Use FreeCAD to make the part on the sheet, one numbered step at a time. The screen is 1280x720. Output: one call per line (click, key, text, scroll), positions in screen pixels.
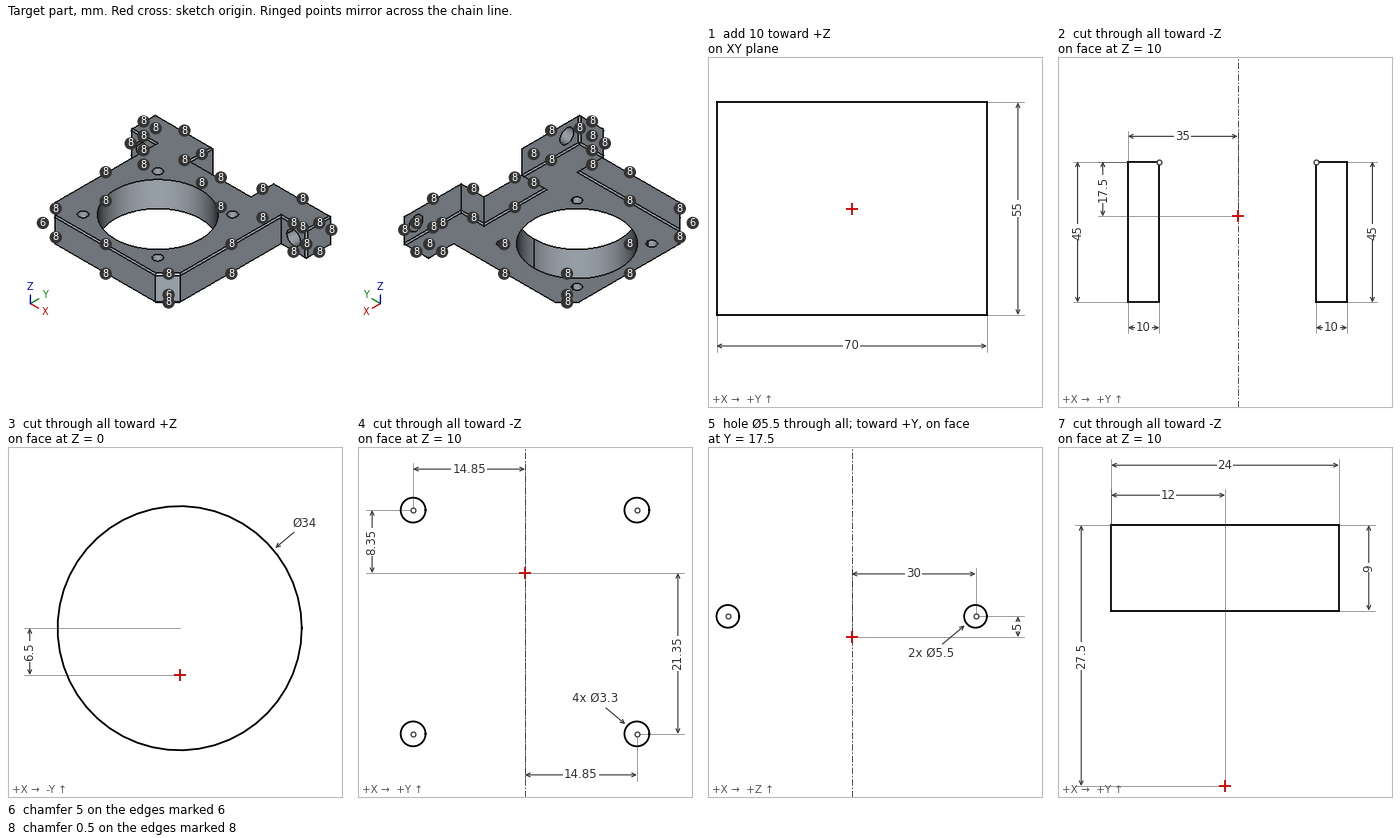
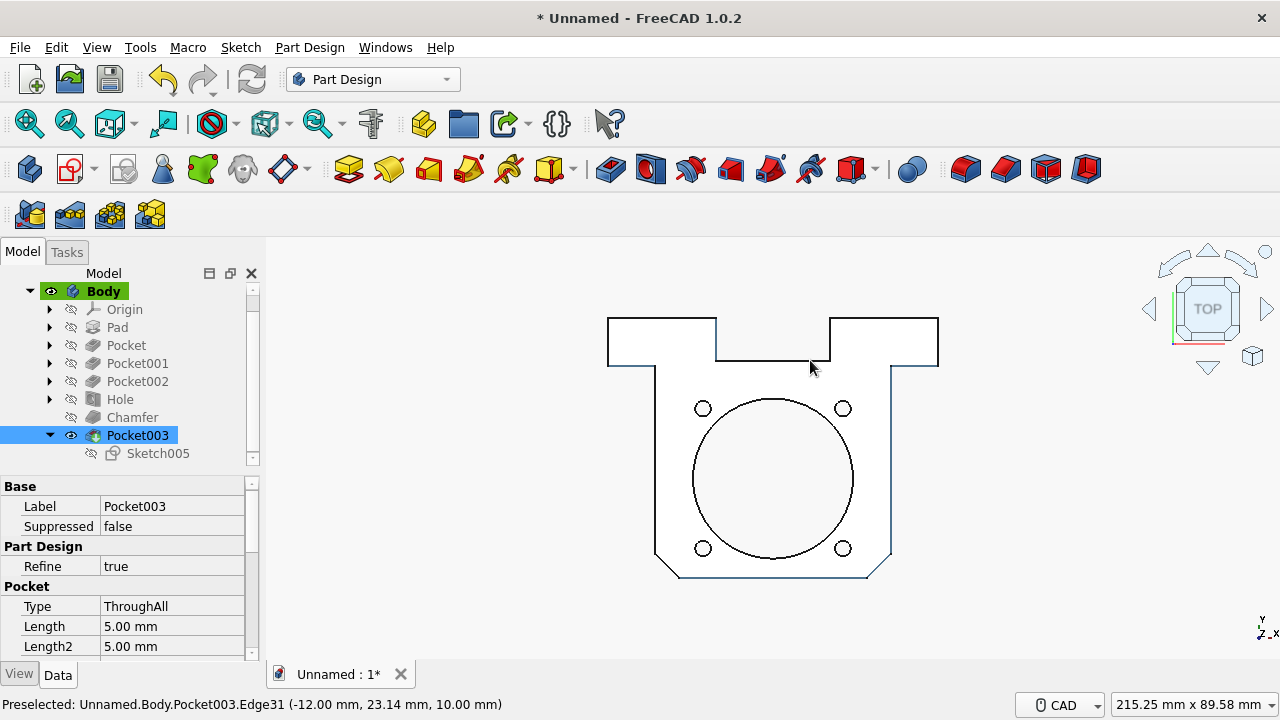
click(773, 360, ctrl)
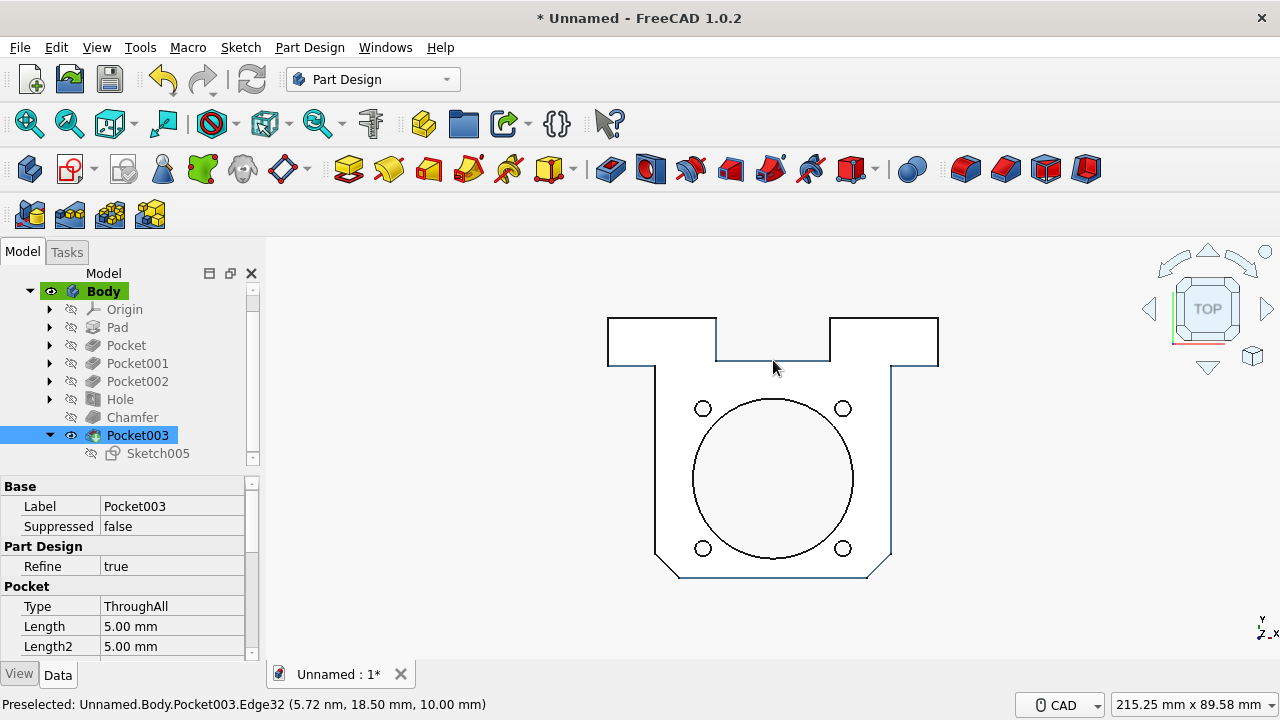
click(830, 339, ctrl)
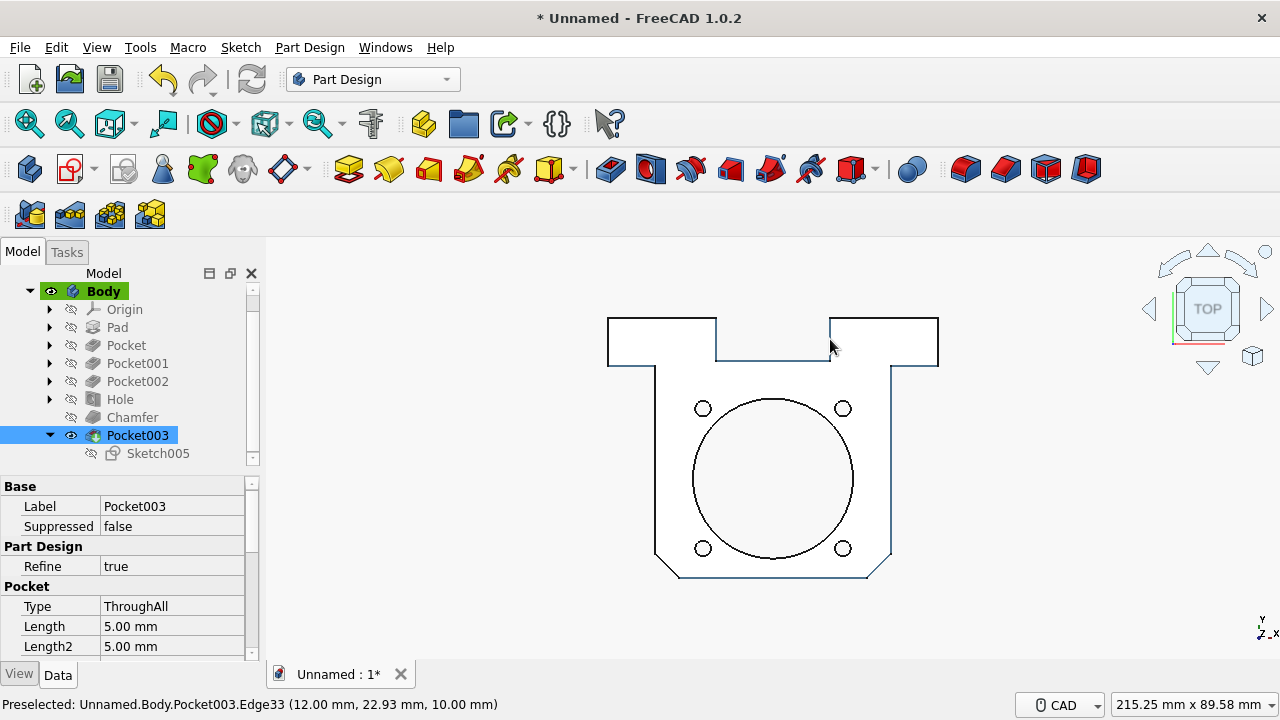
click(884, 317, ctrl)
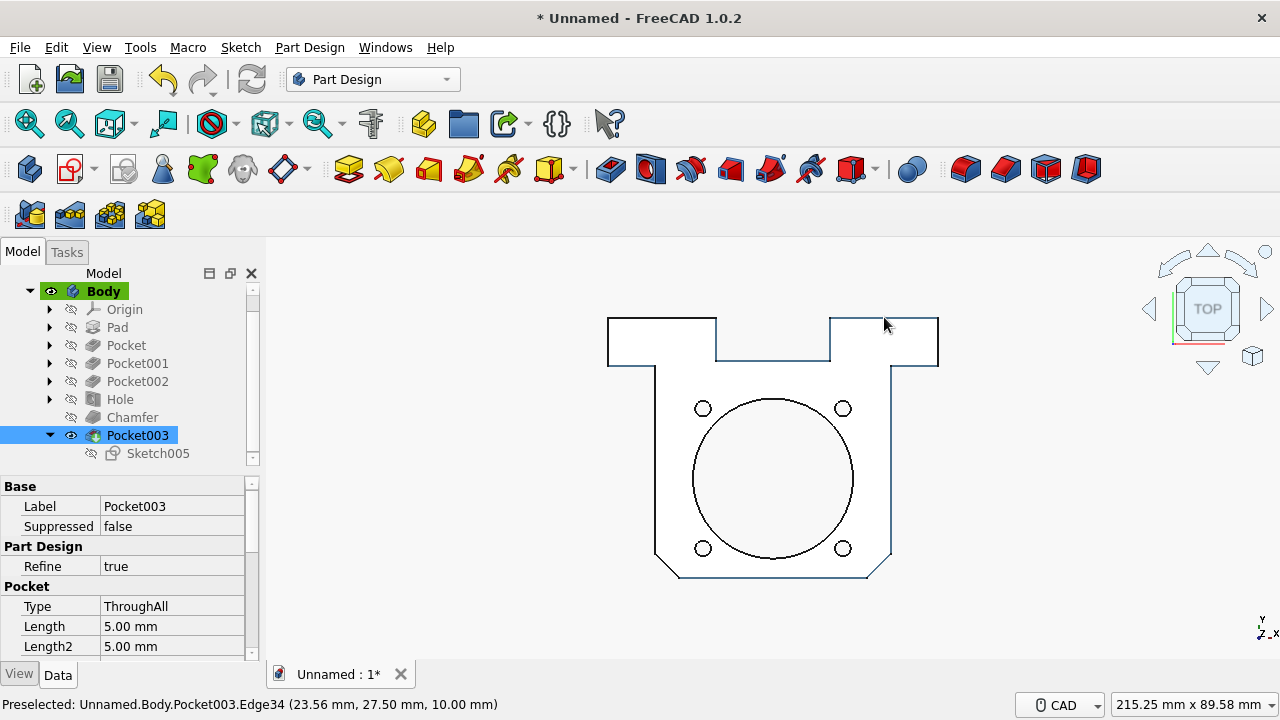
click(655, 459, ctrl)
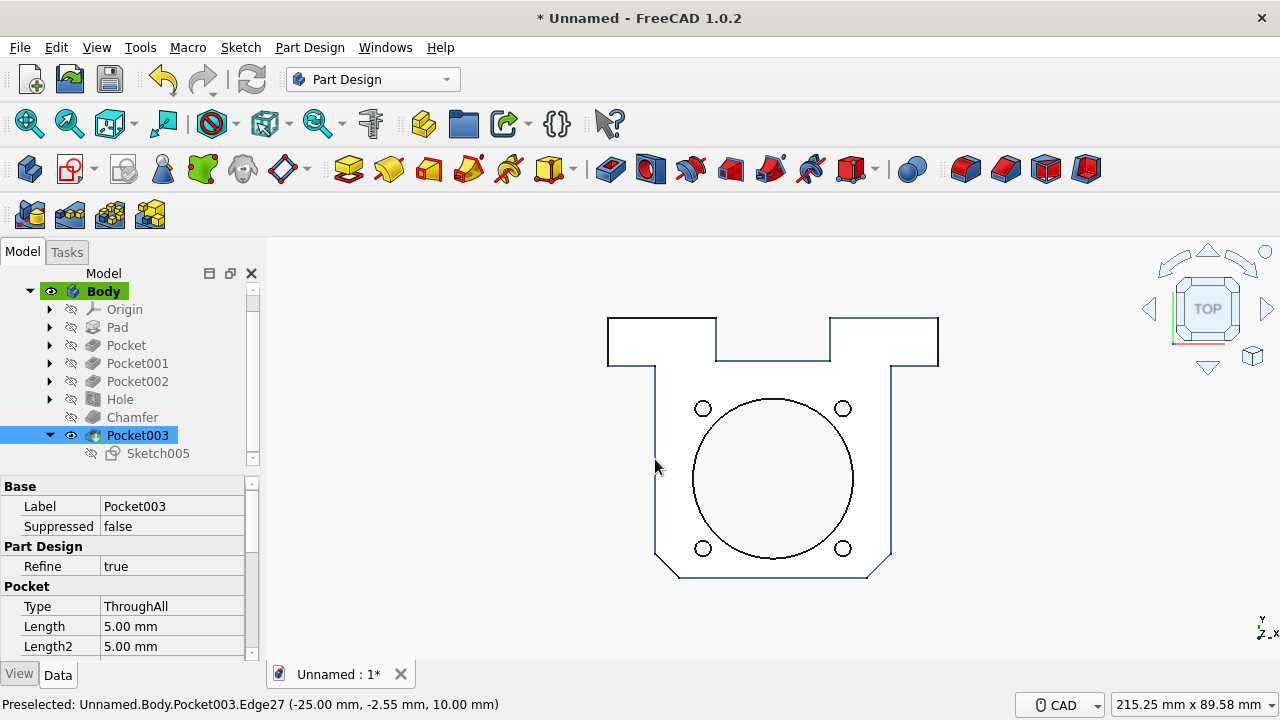
click(667, 565, ctrl)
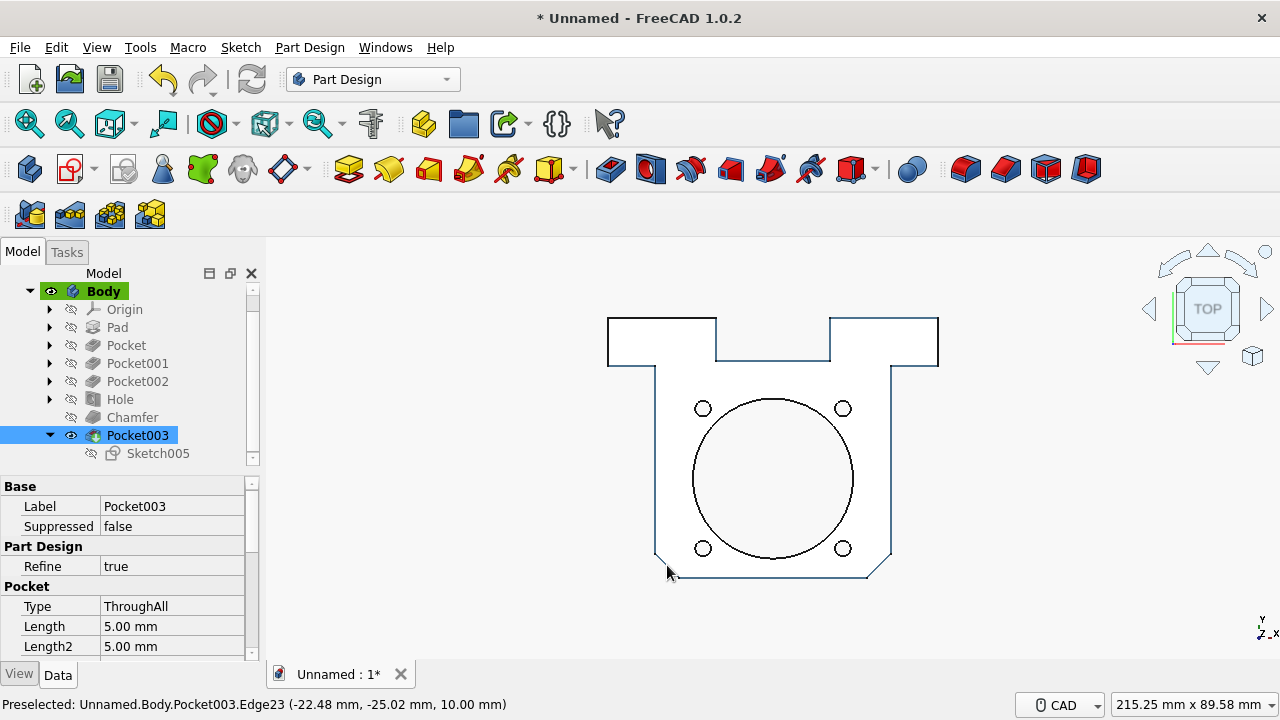
click(662, 317, ctrl)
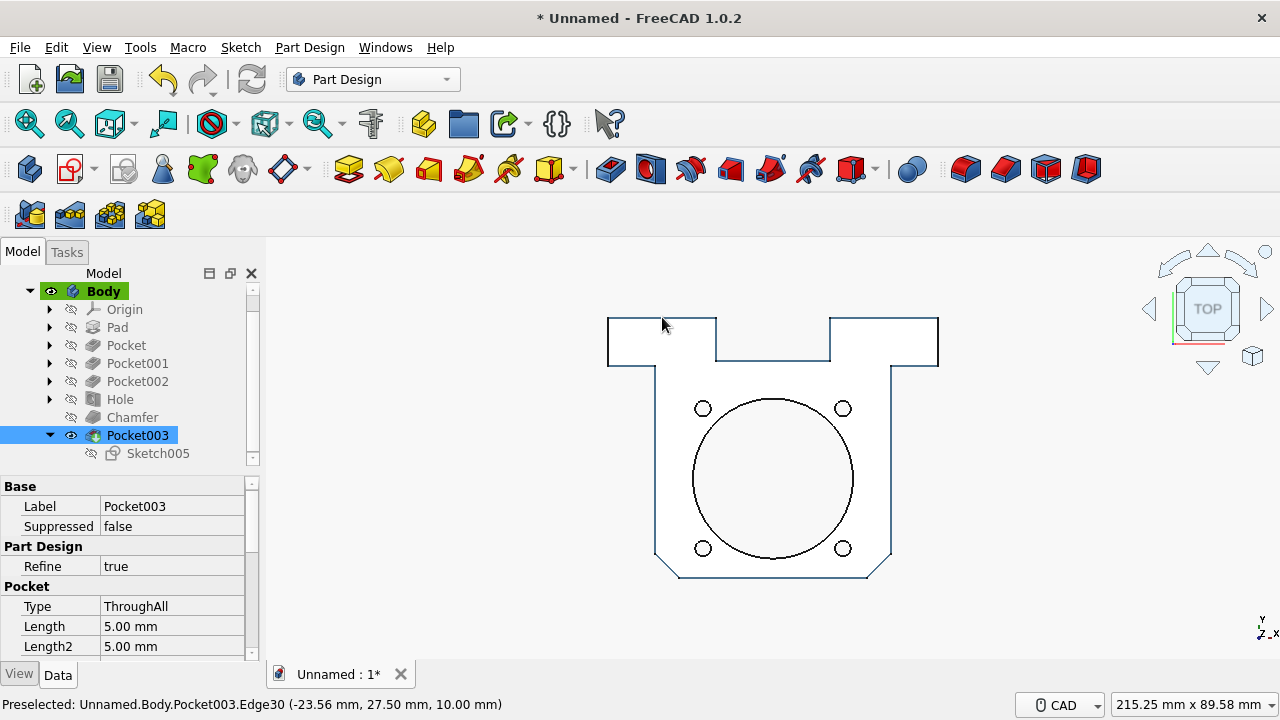
key(0)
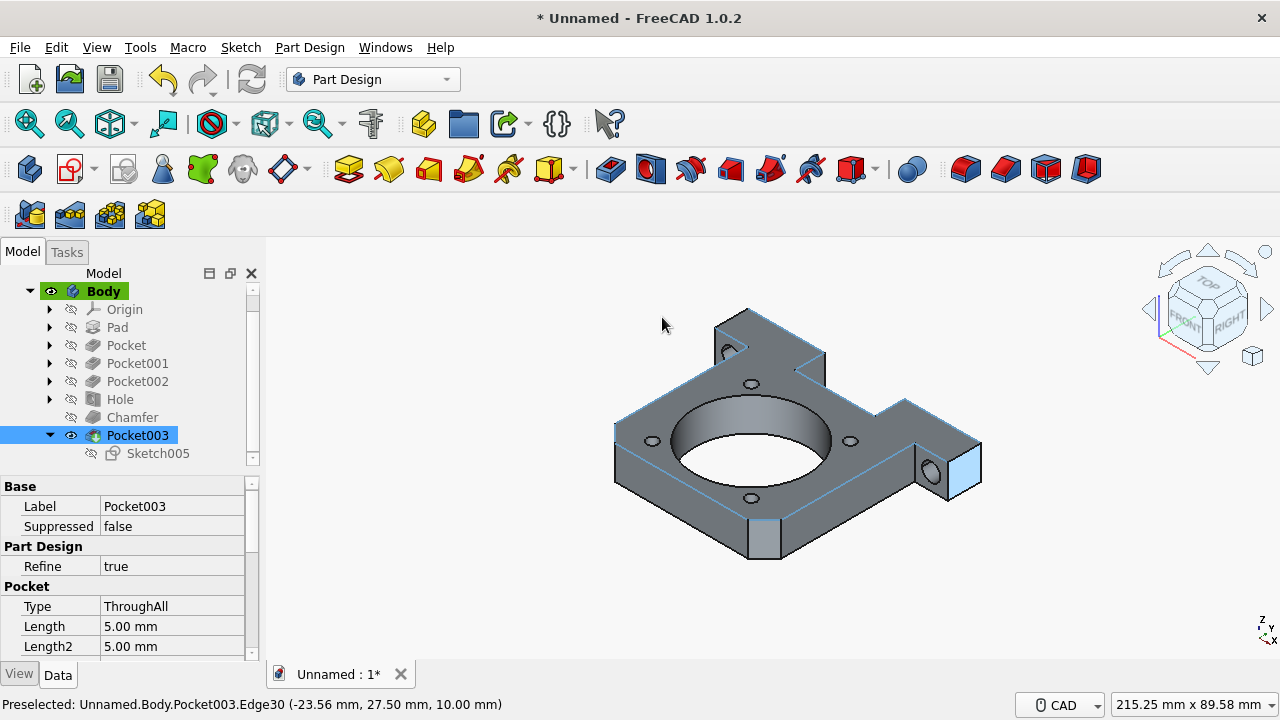
key(1)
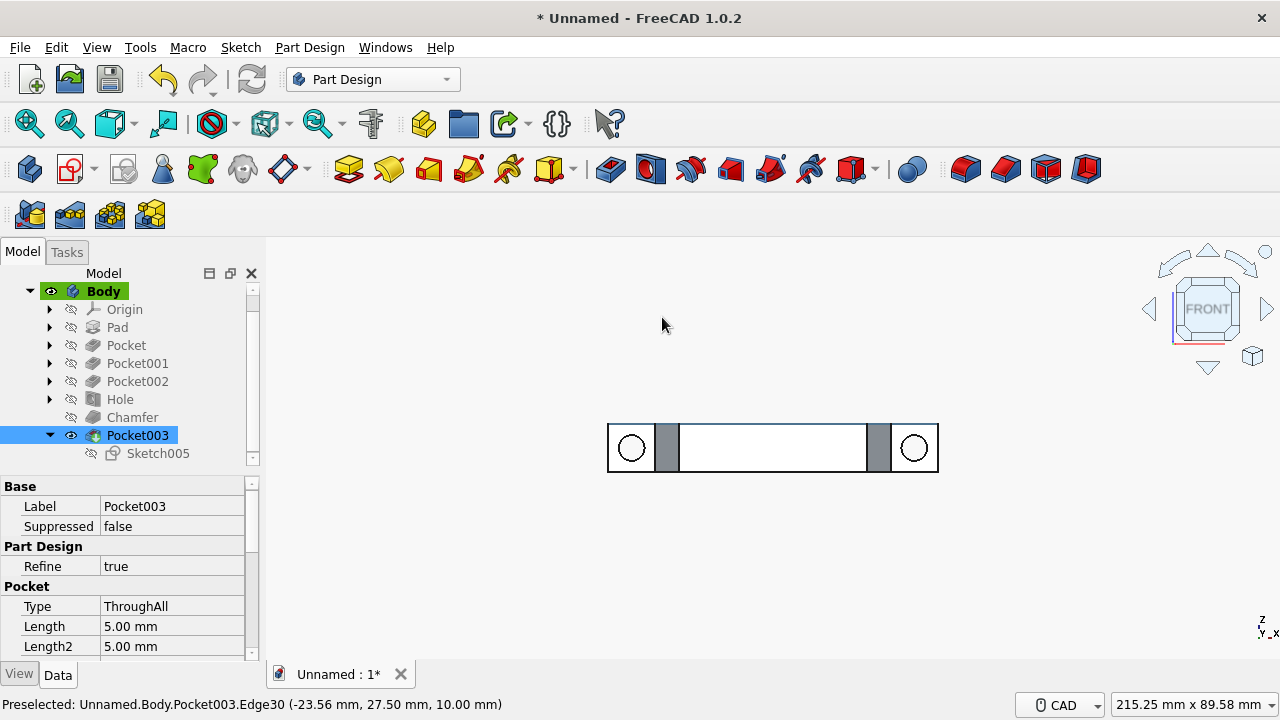
key(v)
key(f)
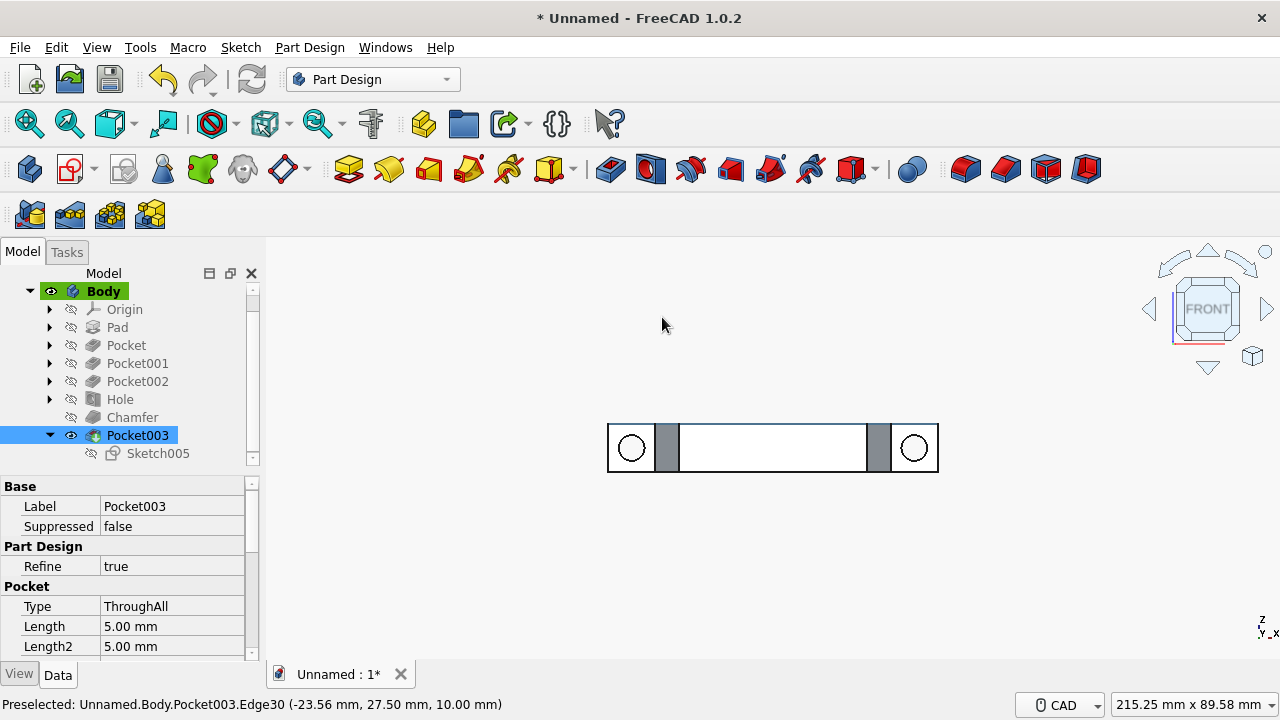
click(632, 471, ctrl)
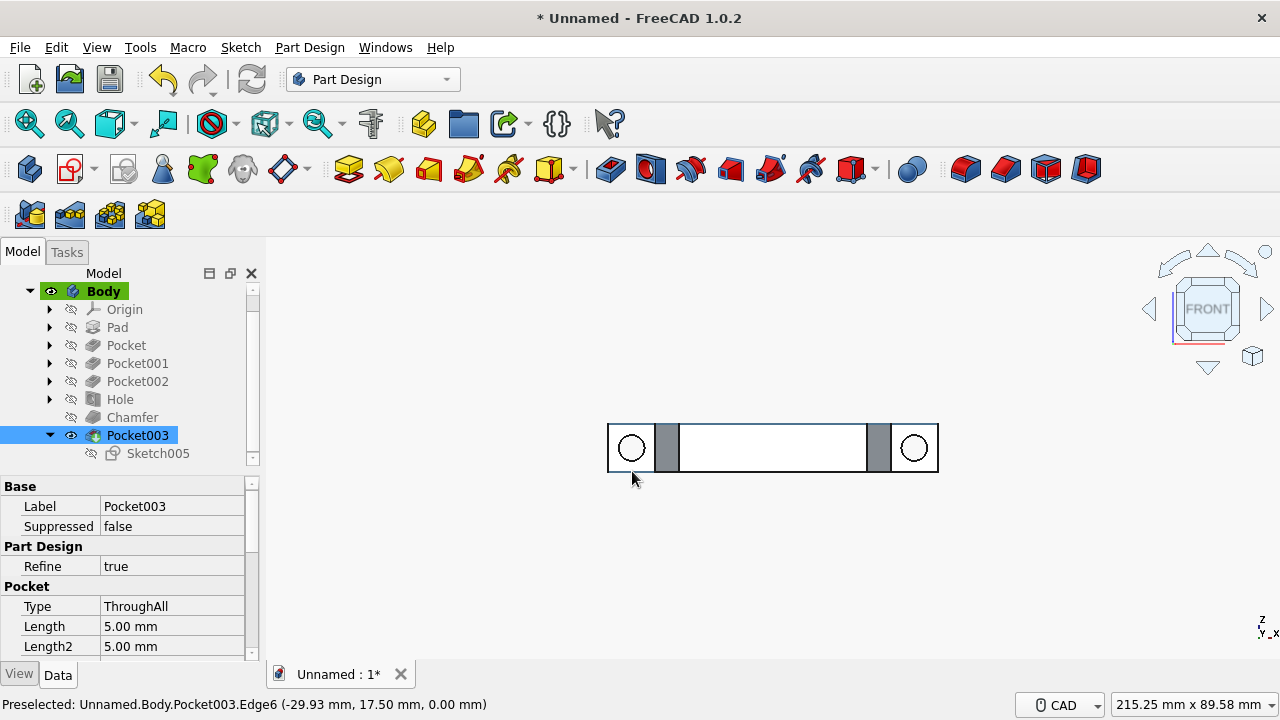
click(914, 471, ctrl)